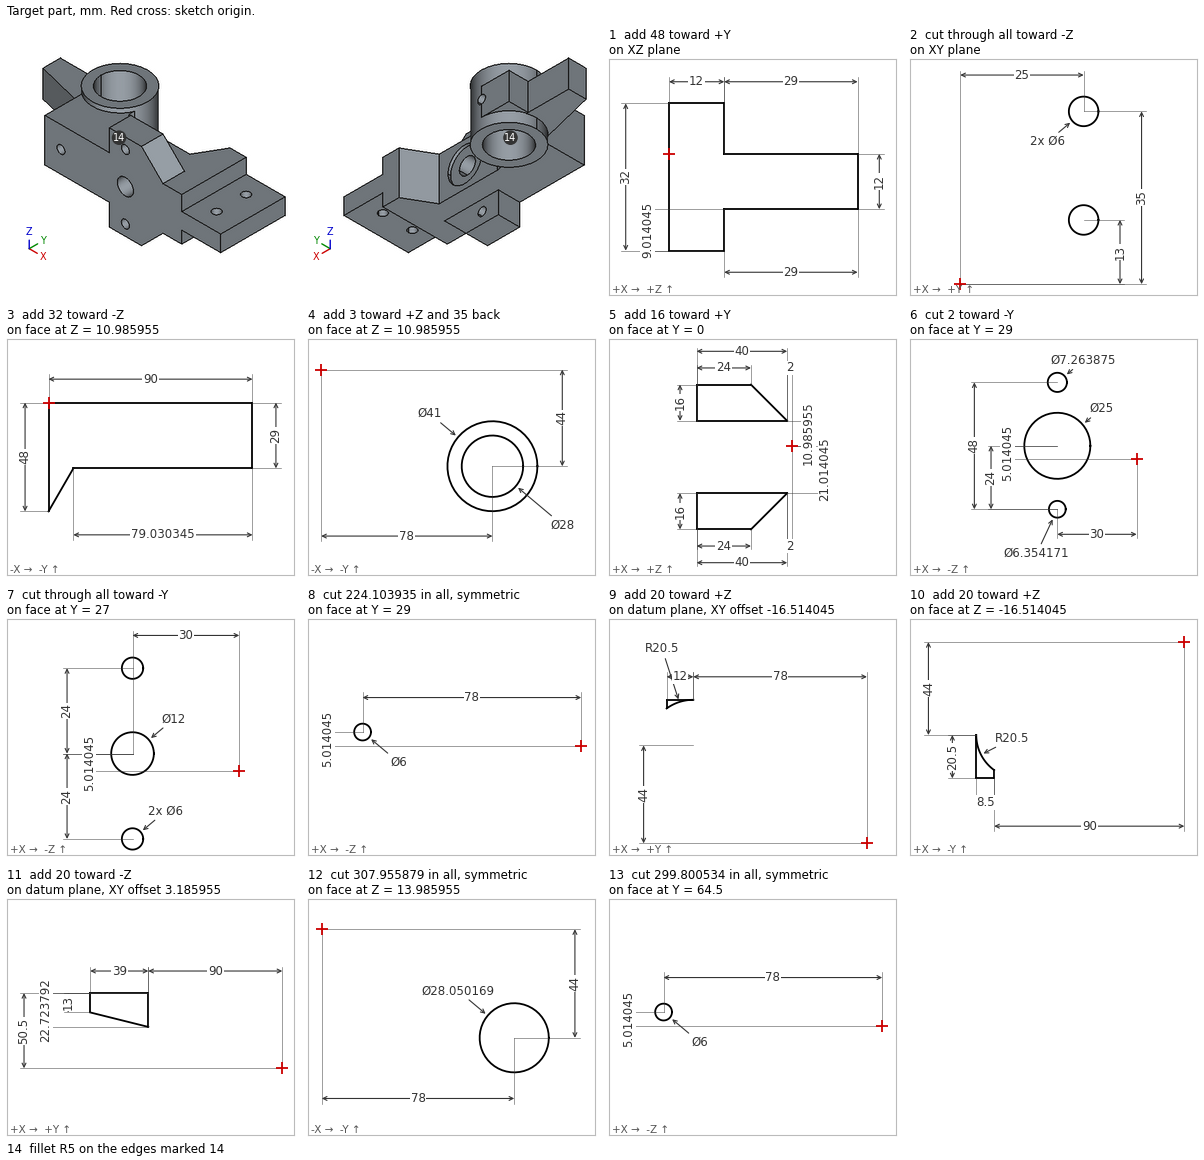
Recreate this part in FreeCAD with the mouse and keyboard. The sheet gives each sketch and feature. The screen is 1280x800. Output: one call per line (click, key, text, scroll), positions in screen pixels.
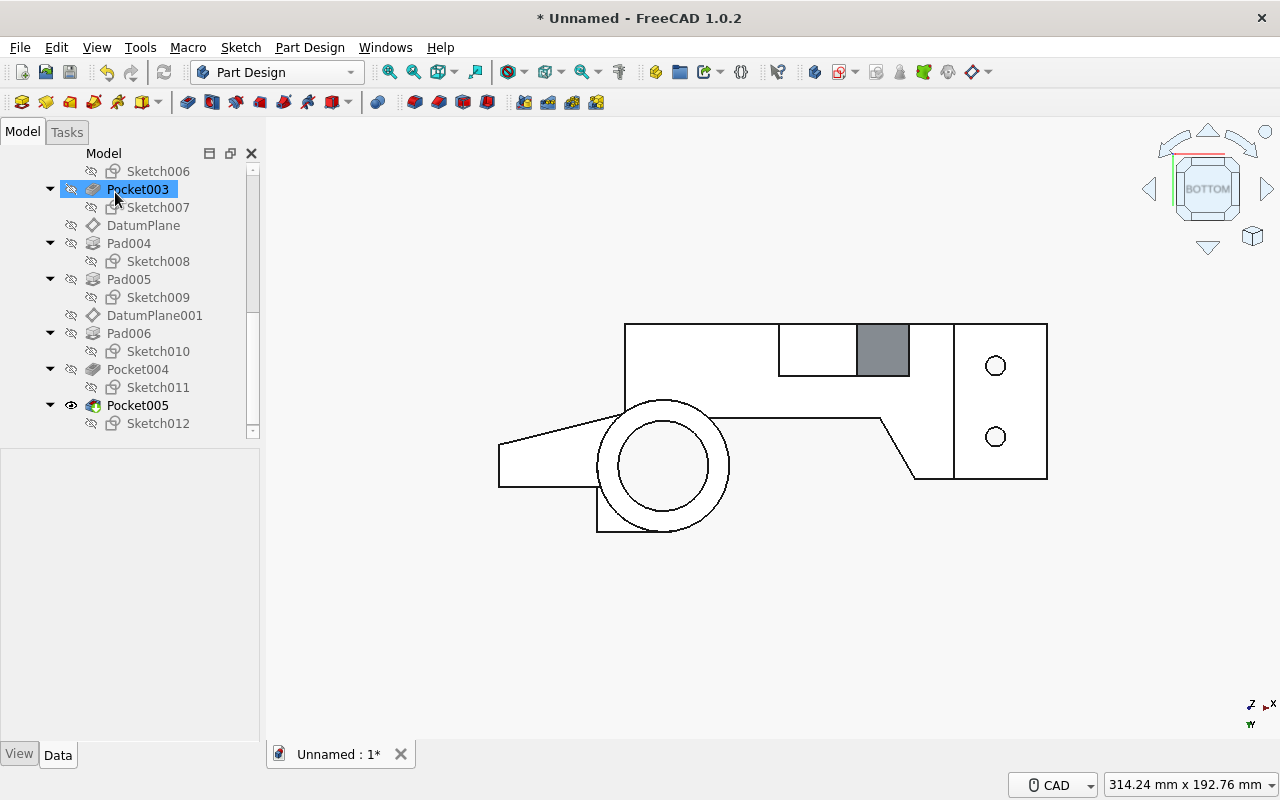
key(4)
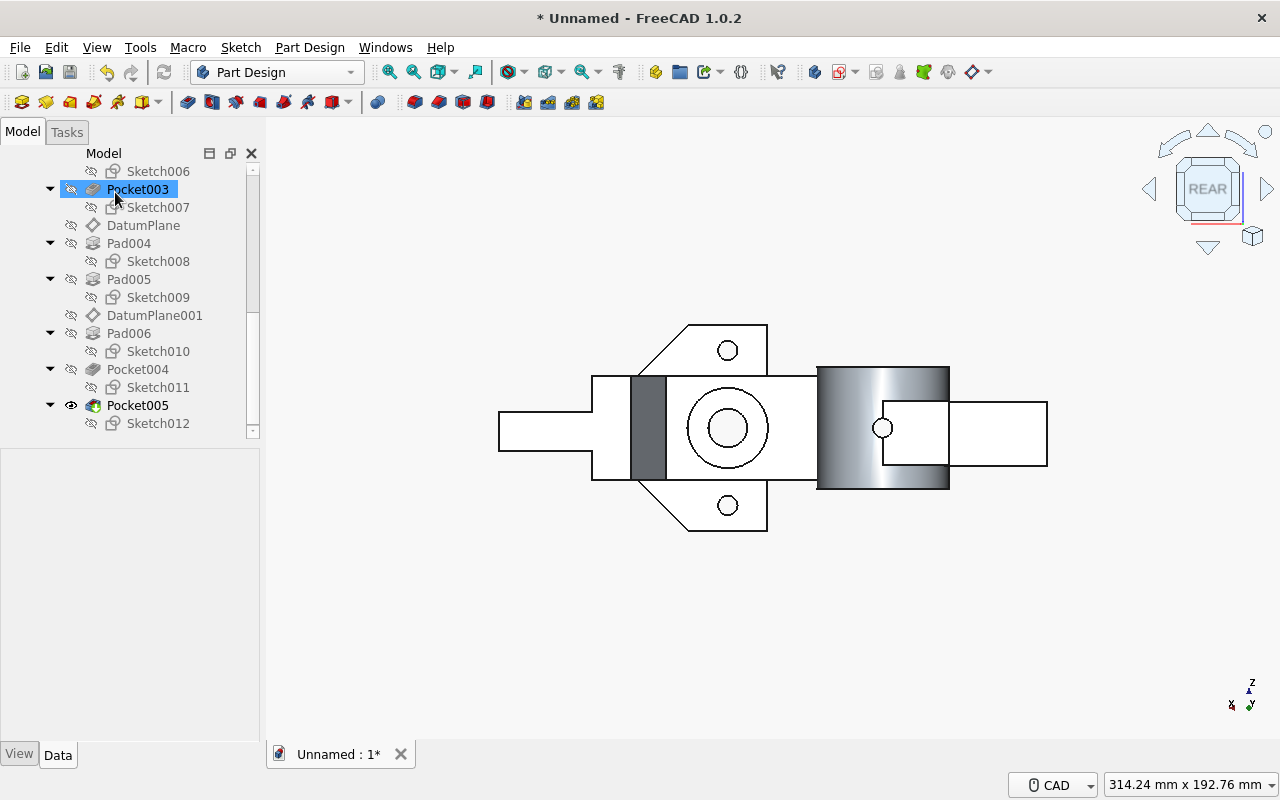
key(6)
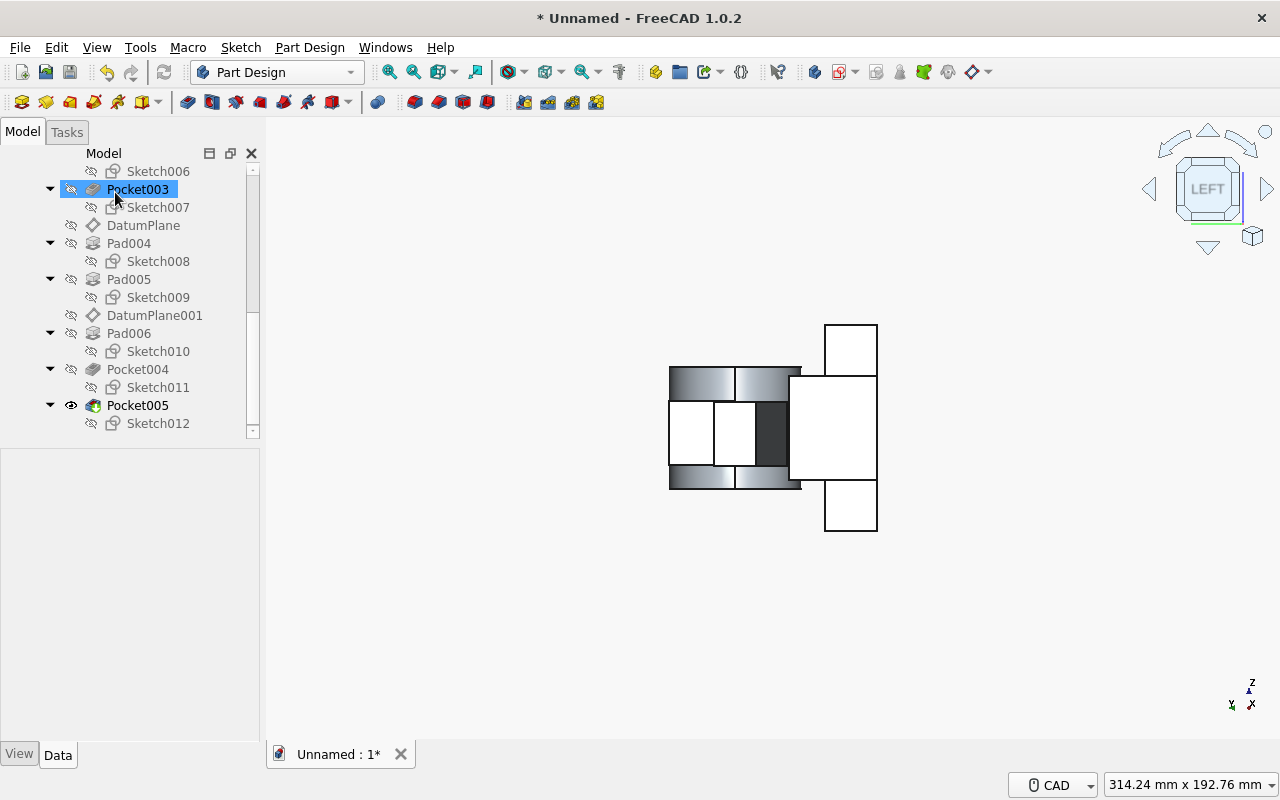
key(v)
key(f)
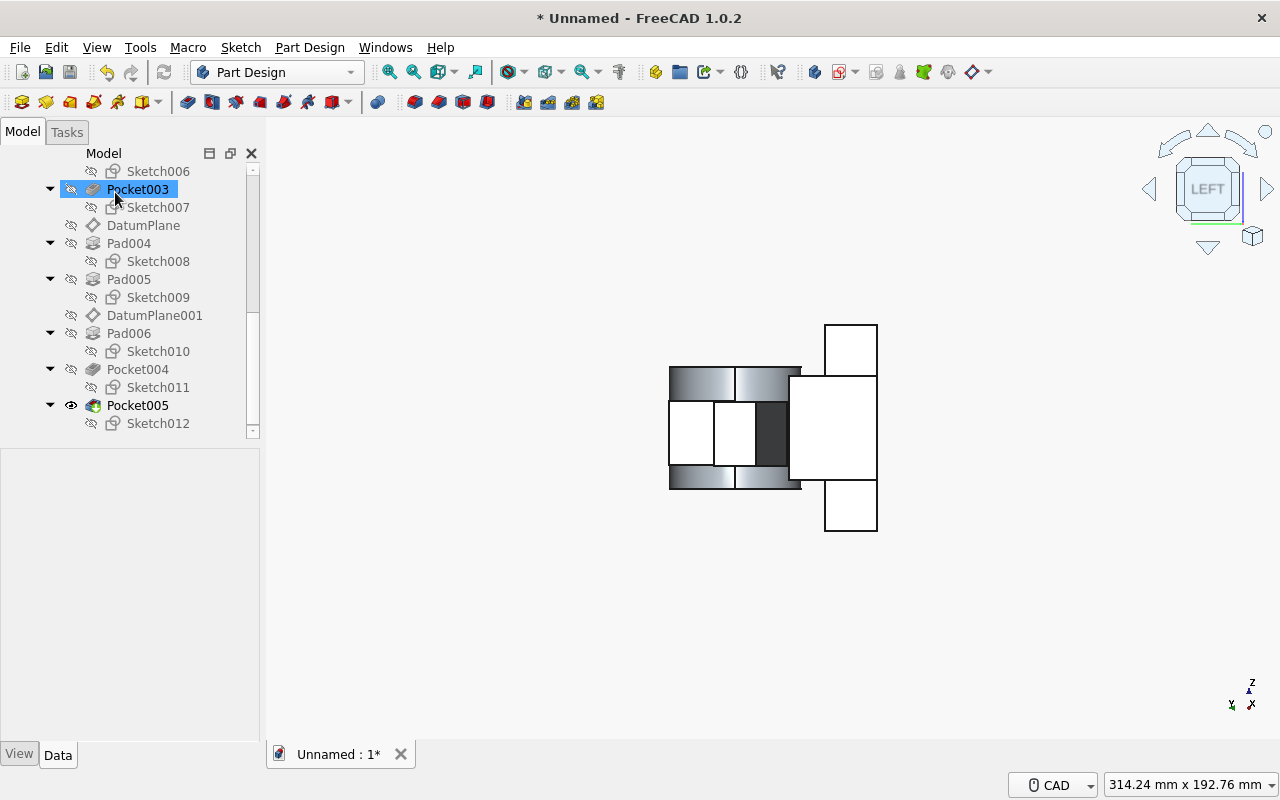
key(v)
key(3)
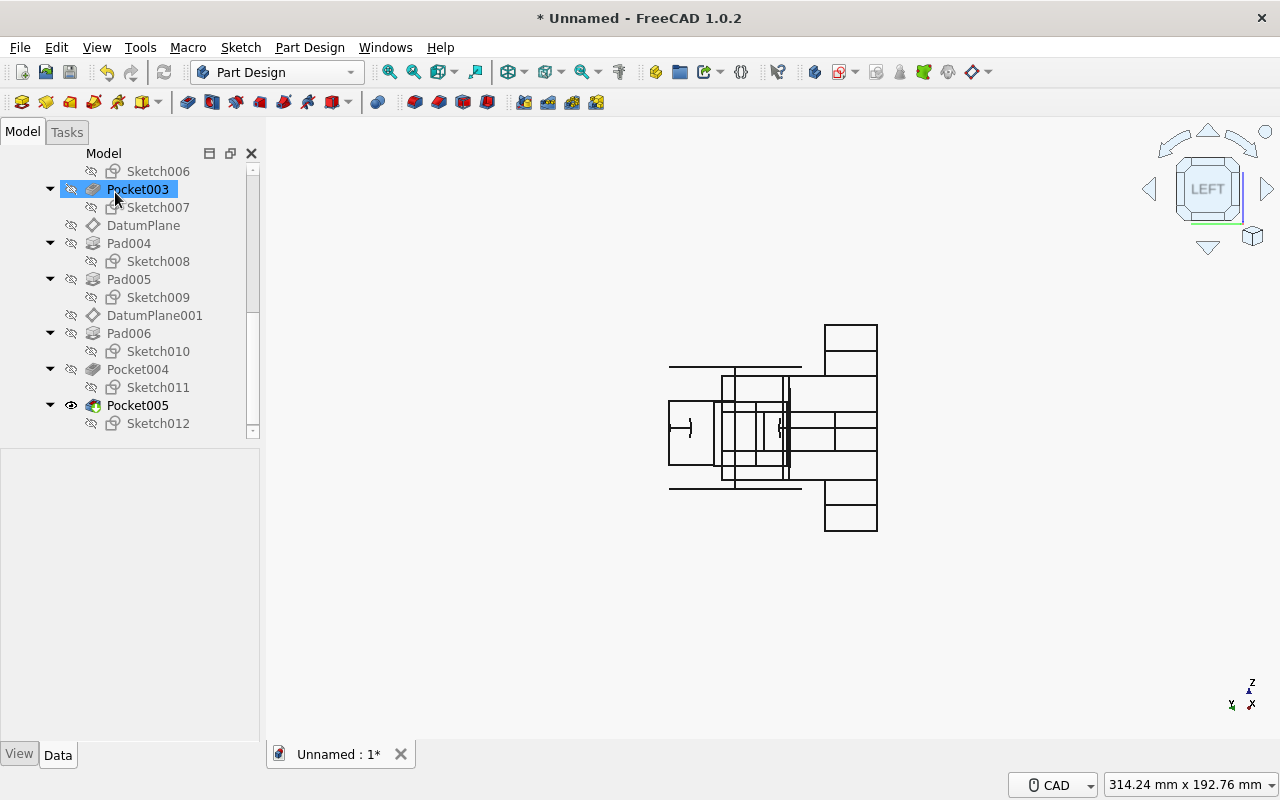
key(0)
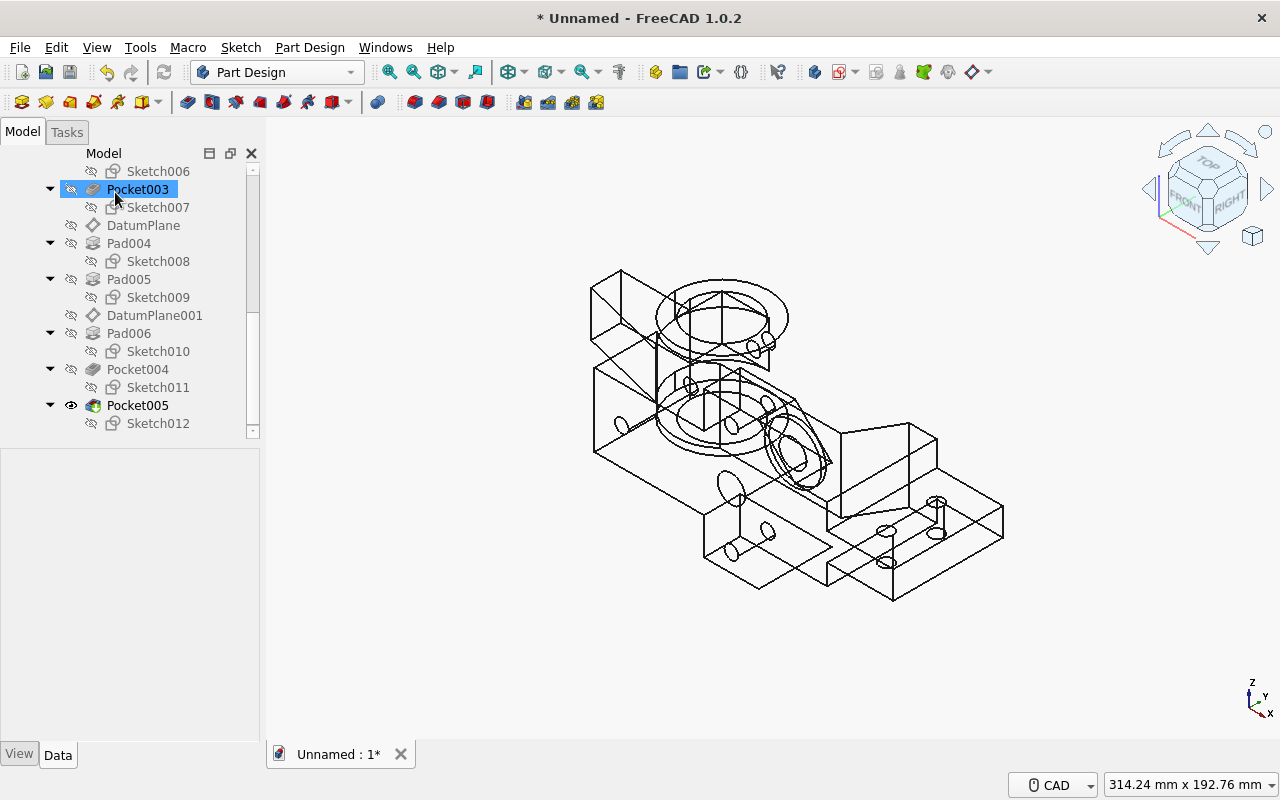
click(720, 405)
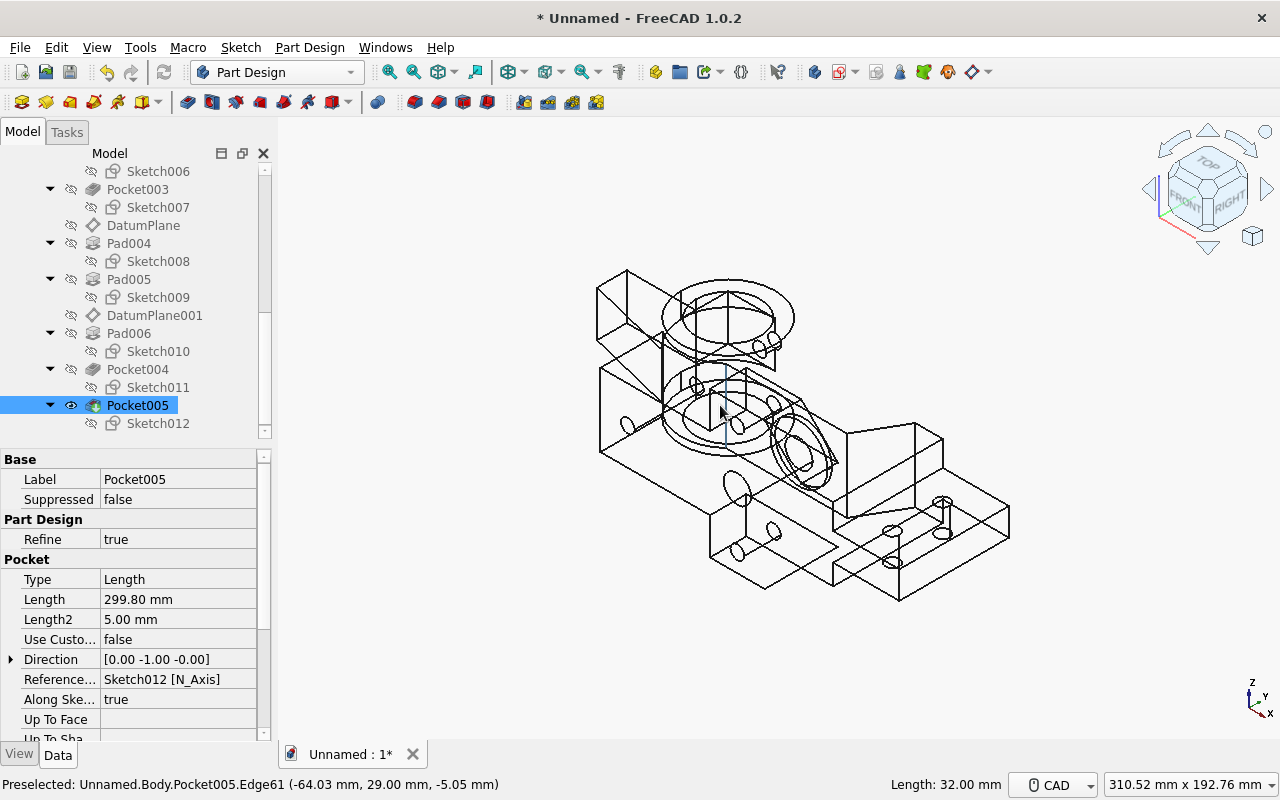
key(v)
key(1)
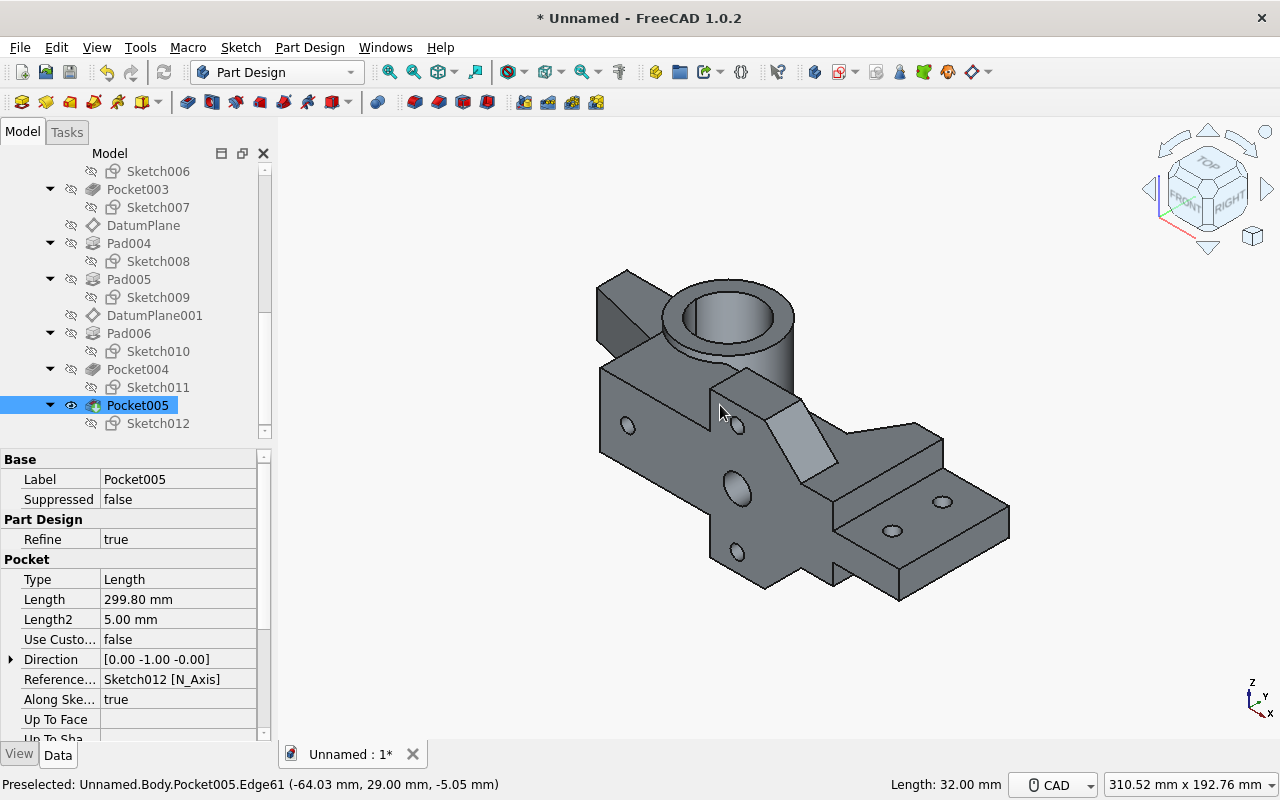
click(416, 102)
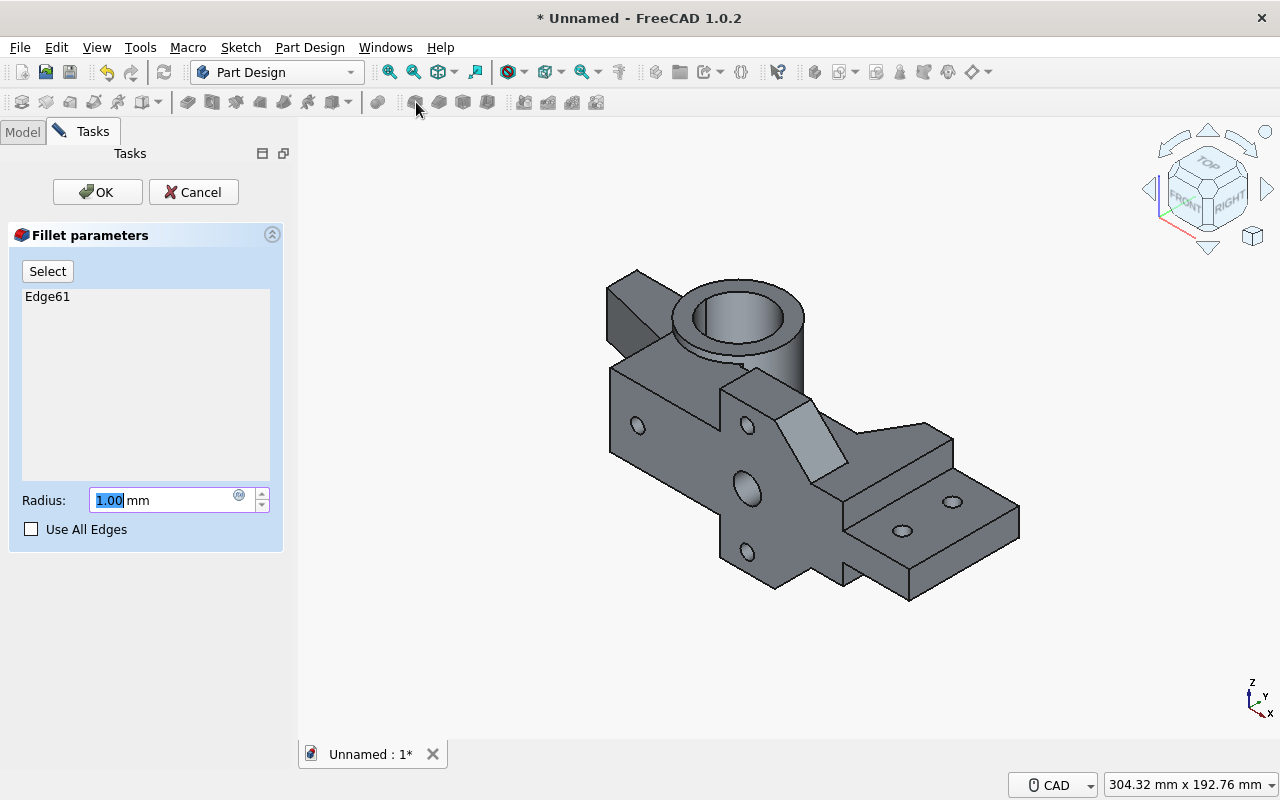
text(5)
key(Tab)